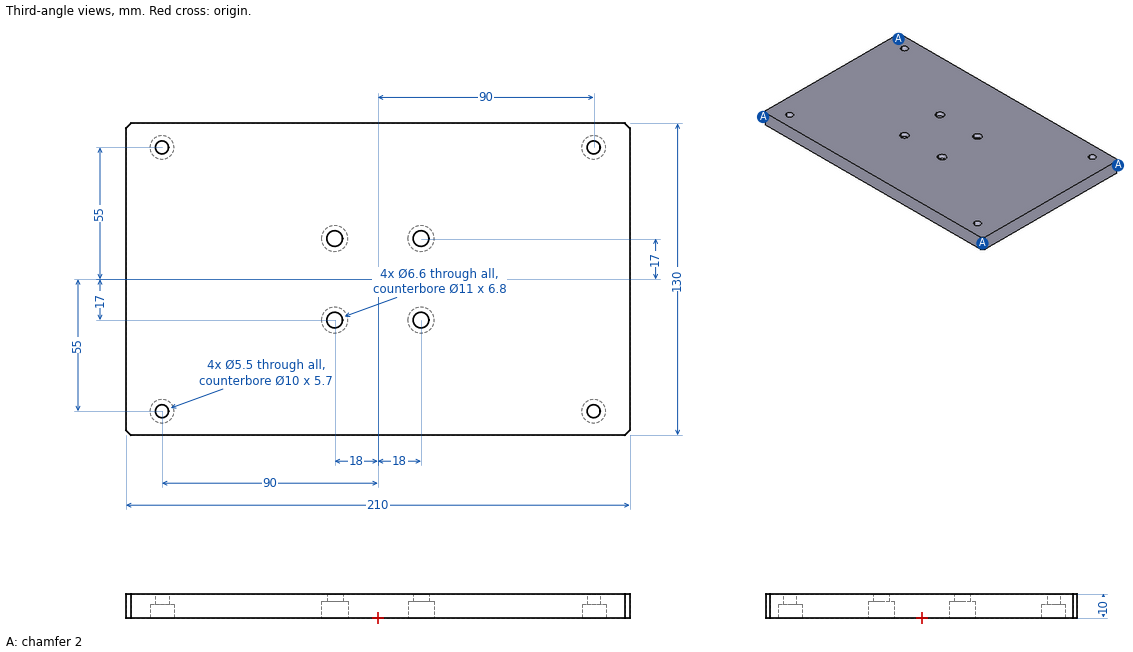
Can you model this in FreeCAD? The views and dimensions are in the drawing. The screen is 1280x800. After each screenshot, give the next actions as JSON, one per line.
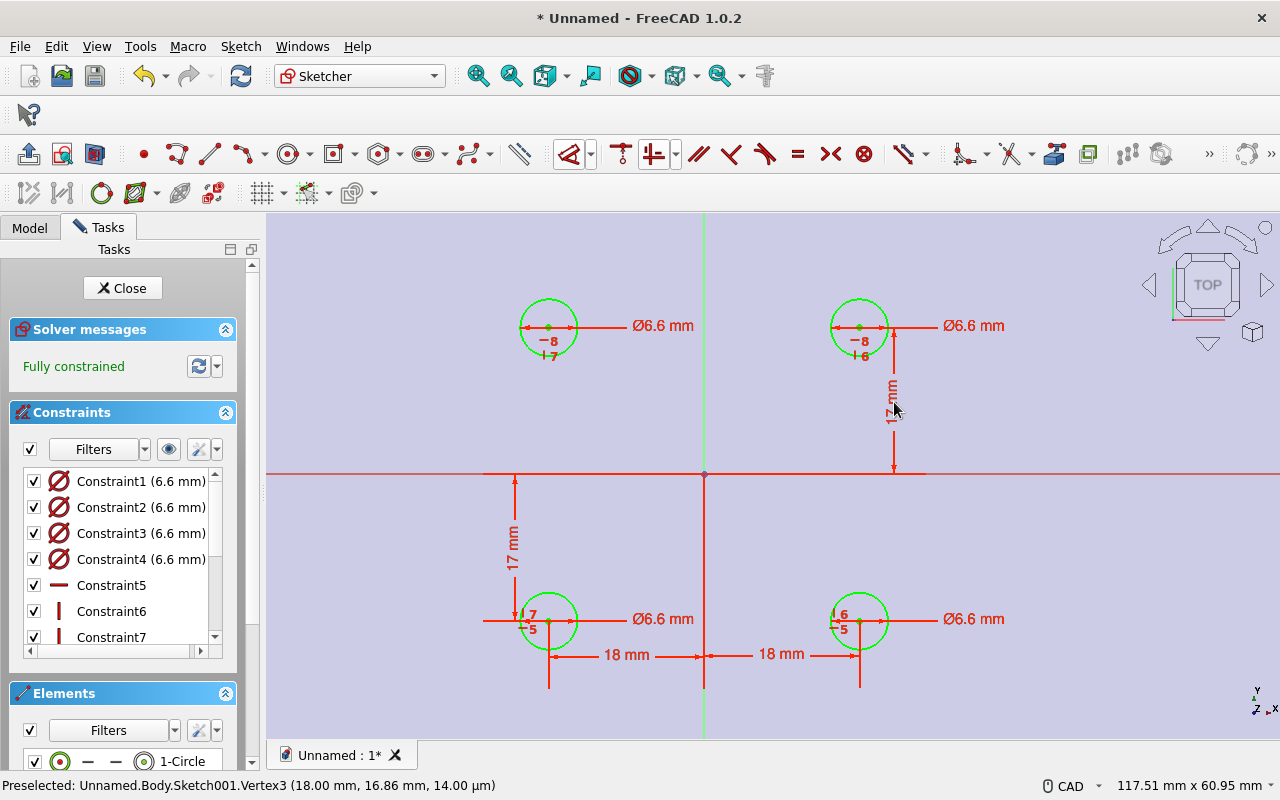
{"action": "left_click", "coordinate": [123, 288]}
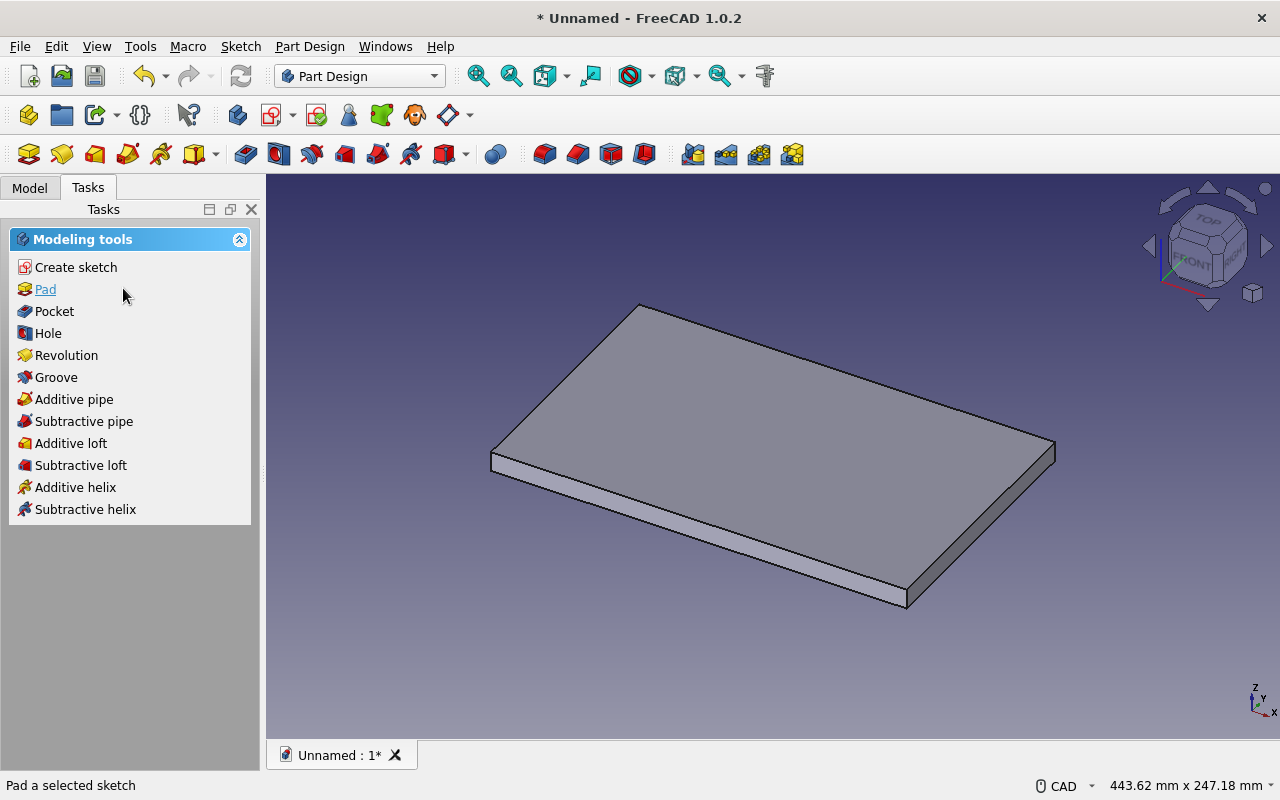
{"action": "left_click", "coordinate": [279, 154]}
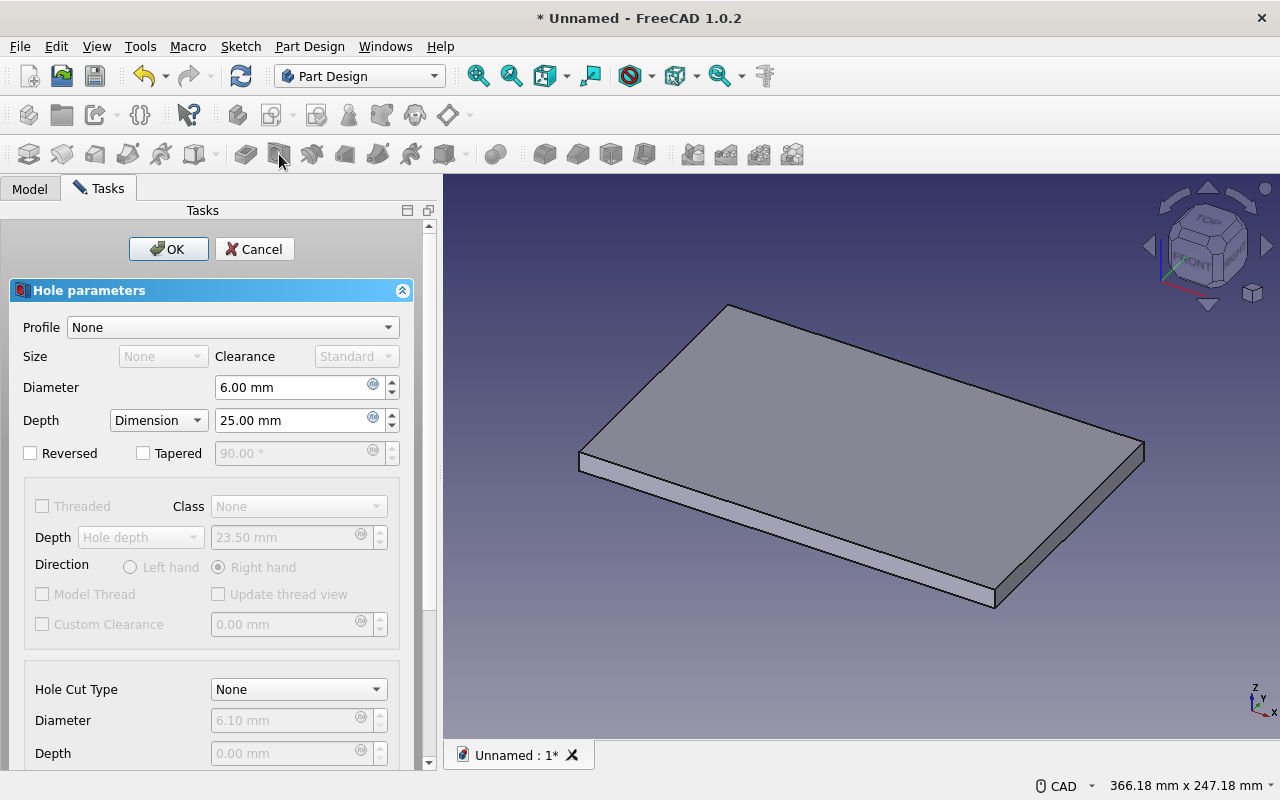
{"action": "triple_click", "coordinate": [300, 388]}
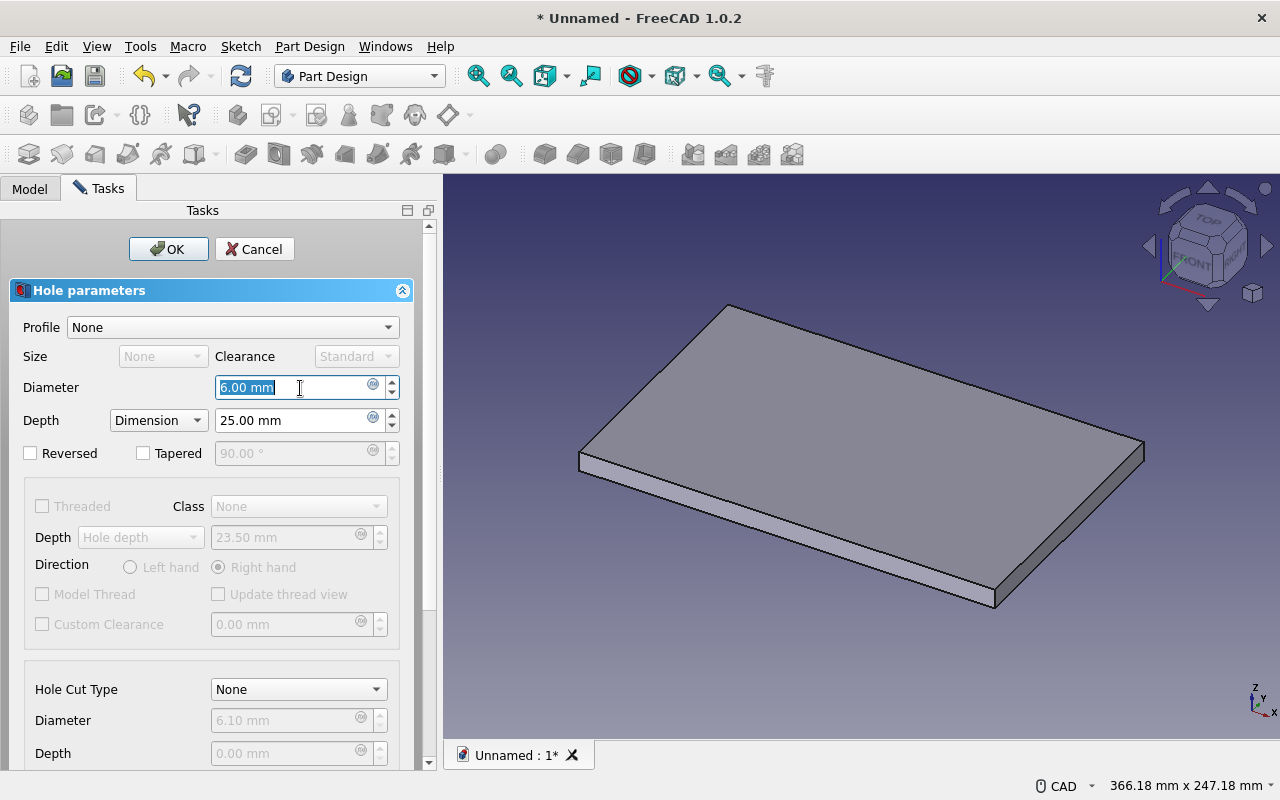
{"action": "type", "text": "6.6"}
{"action": "key", "text": "Tab"}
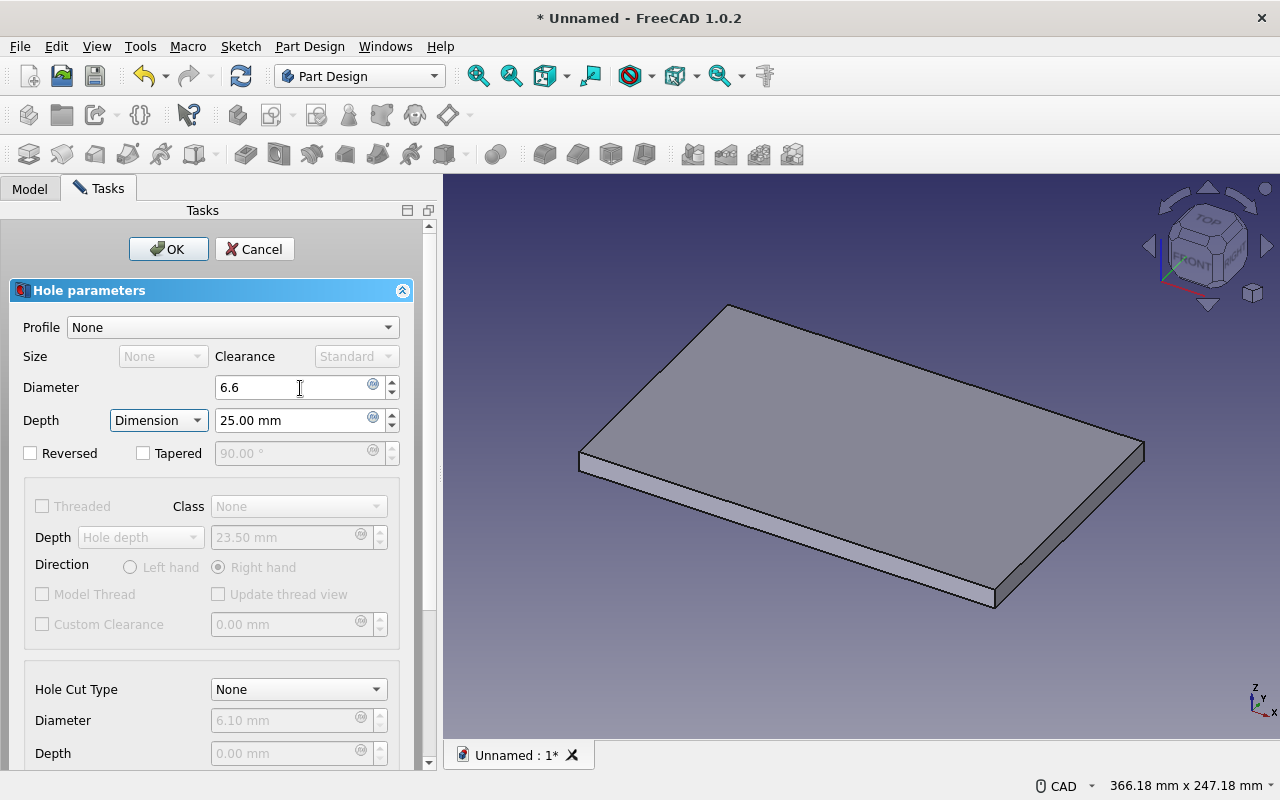
{"action": "left_click", "coordinate": [160, 420]}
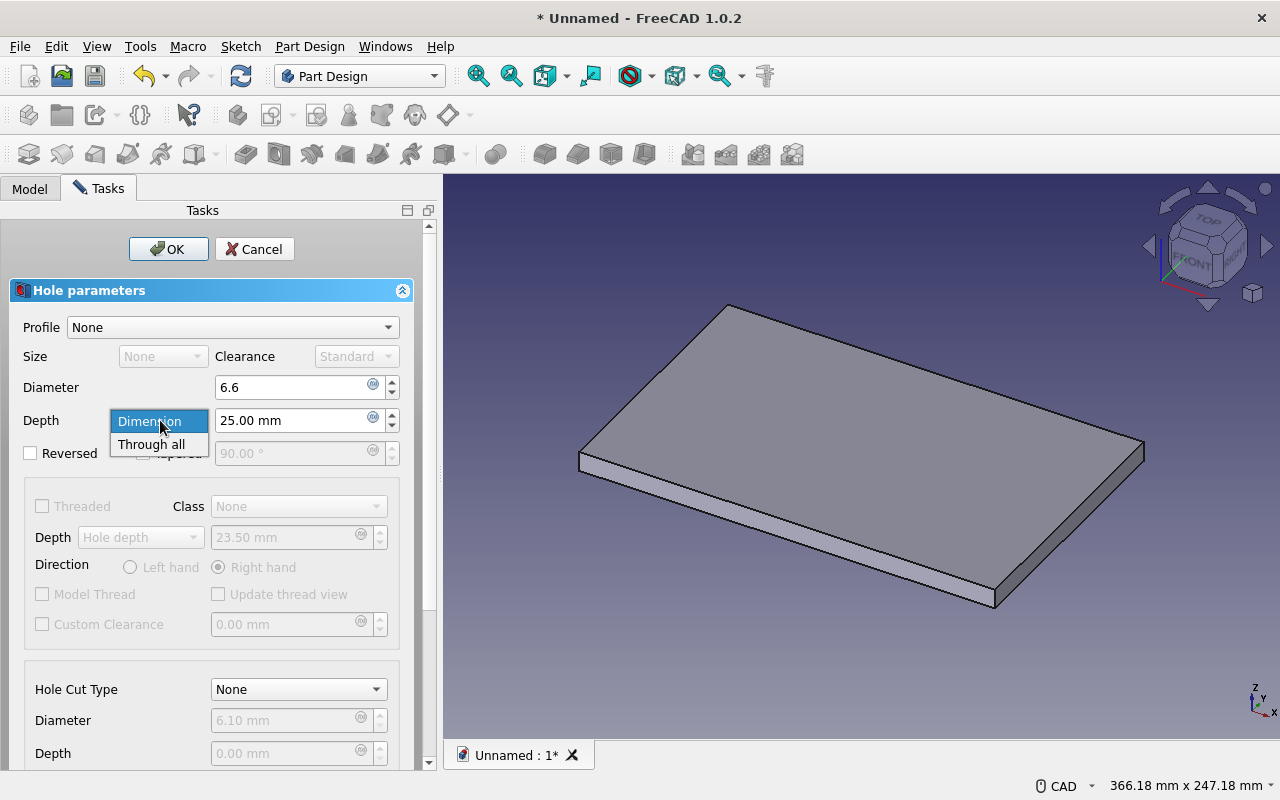
{"action": "left_click", "coordinate": [158, 444]}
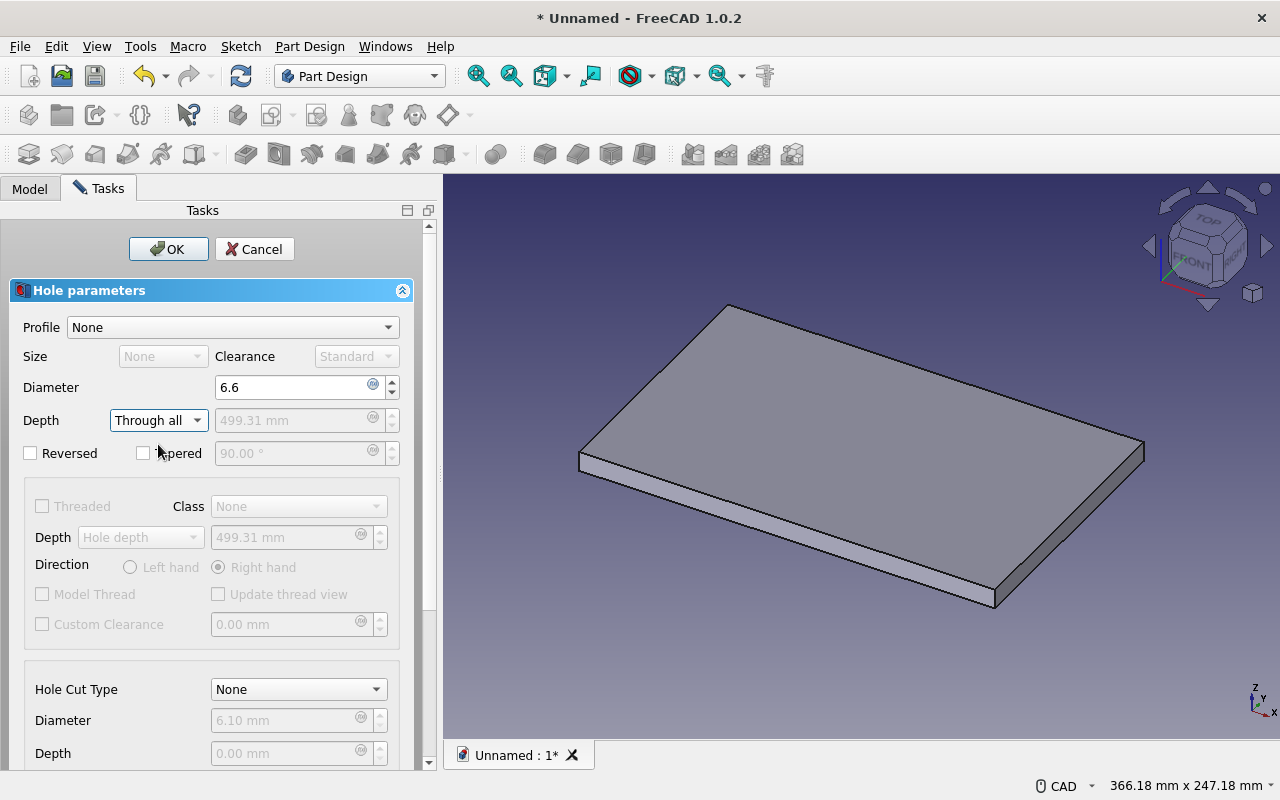
{"action": "left_click", "coordinate": [31, 453]}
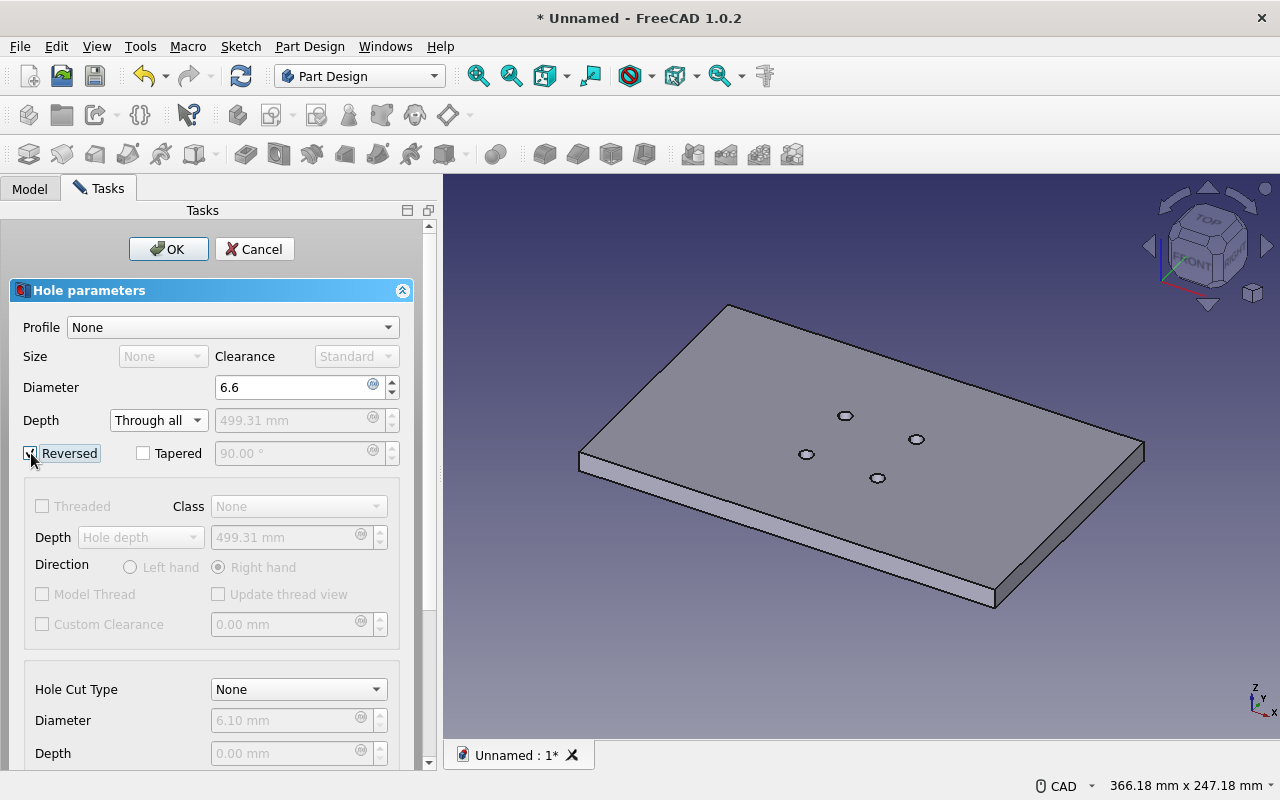
{"action": "left_click", "coordinate": [300, 690]}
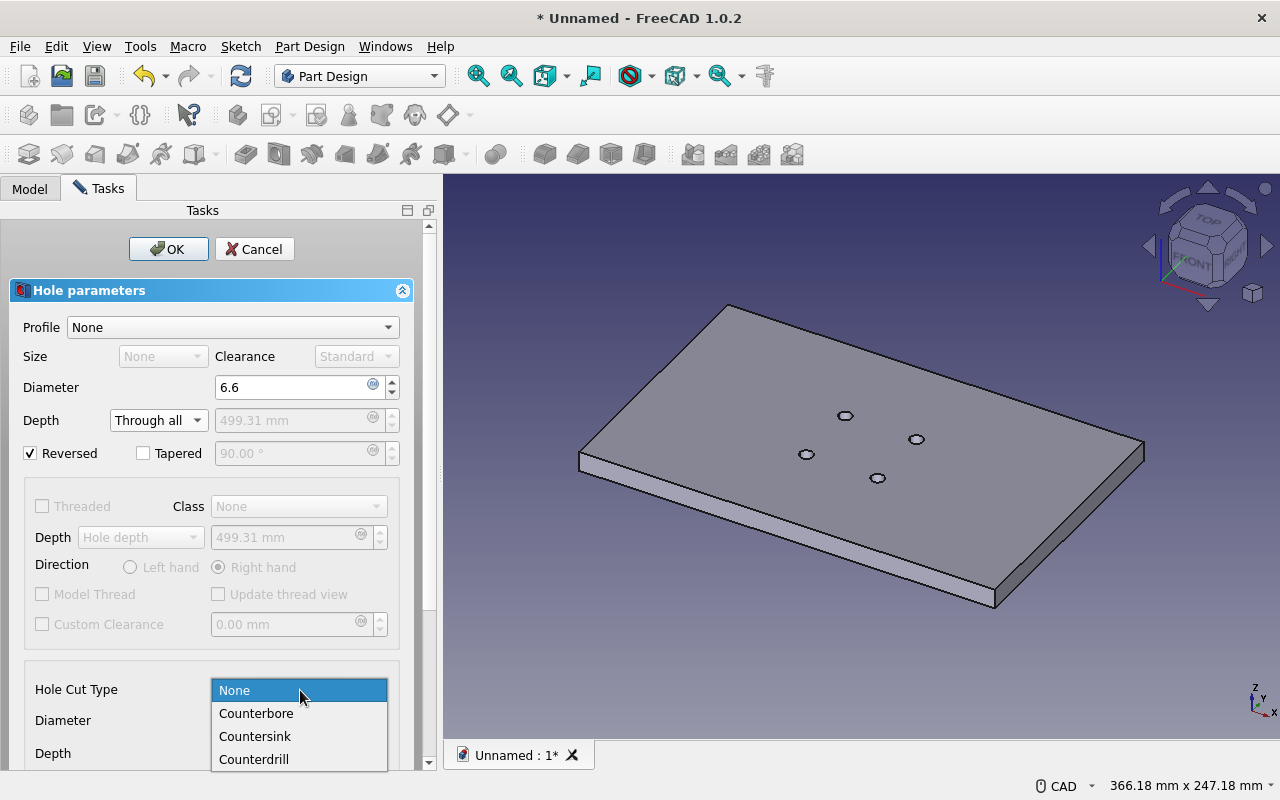
{"action": "left_click", "coordinate": [298, 714]}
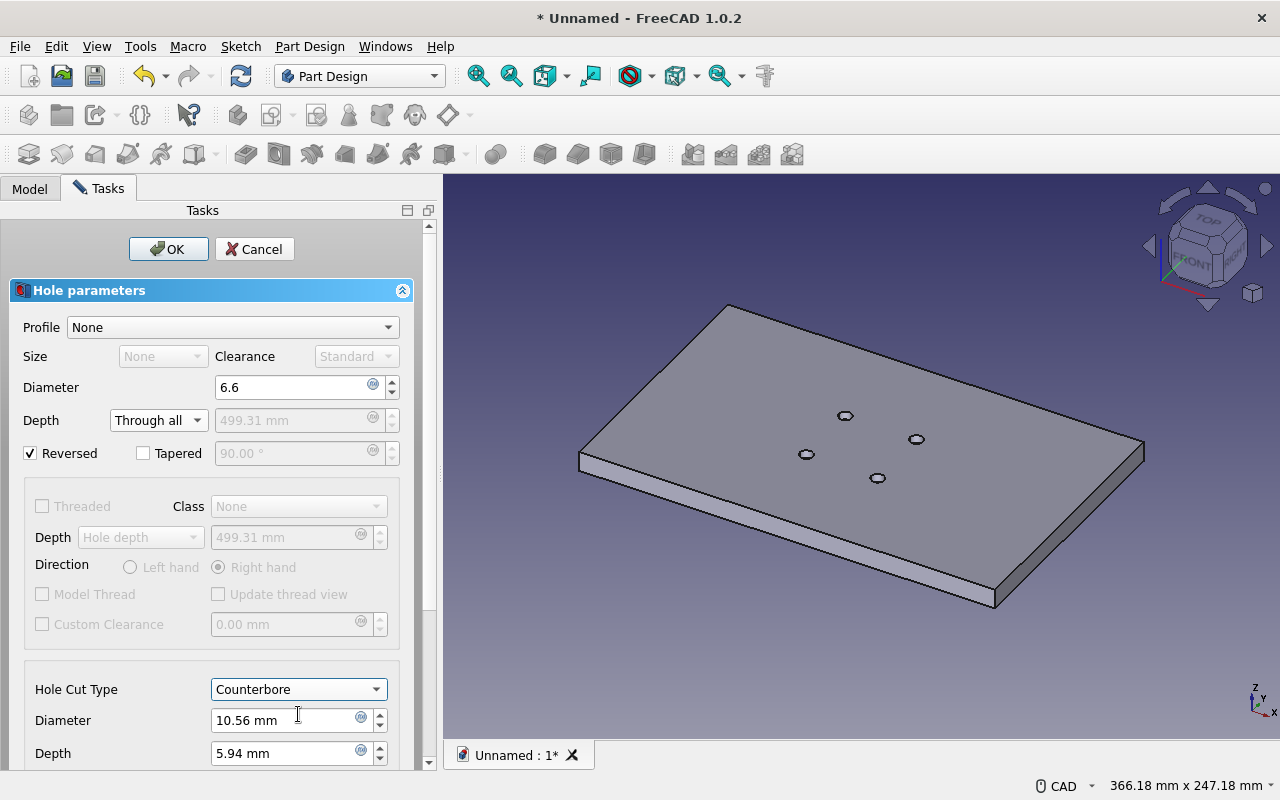
{"action": "triple_click", "coordinate": [292, 720]}